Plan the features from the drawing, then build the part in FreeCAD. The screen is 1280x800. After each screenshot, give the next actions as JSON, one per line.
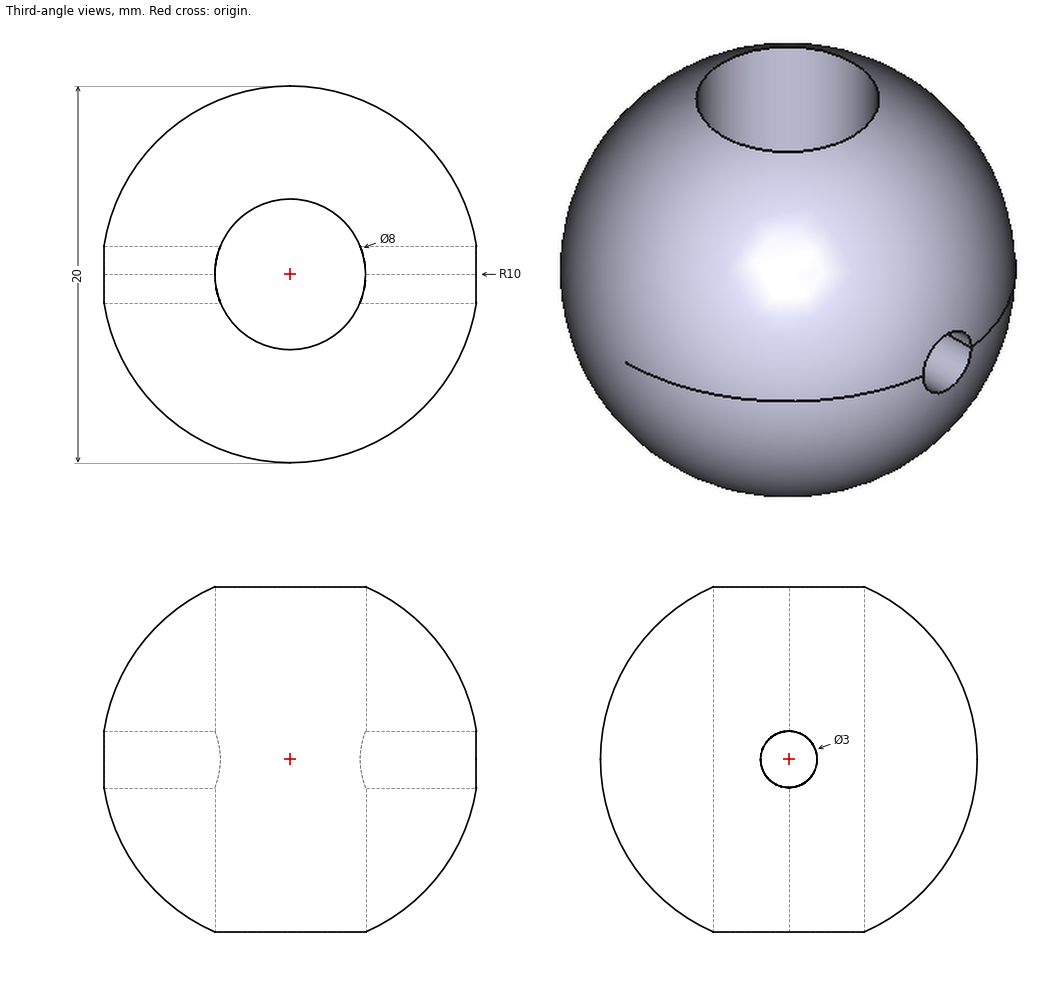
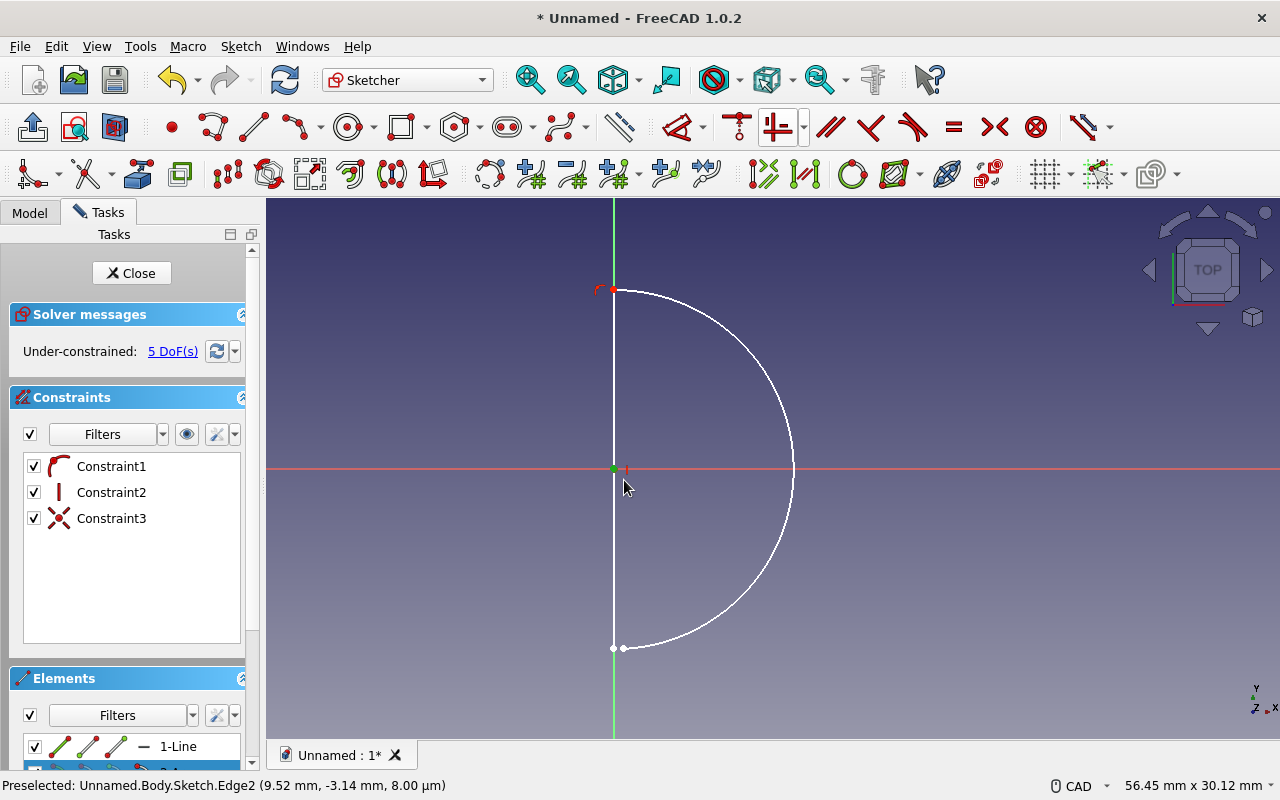
{"action": "left_click", "coordinate": [737, 128]}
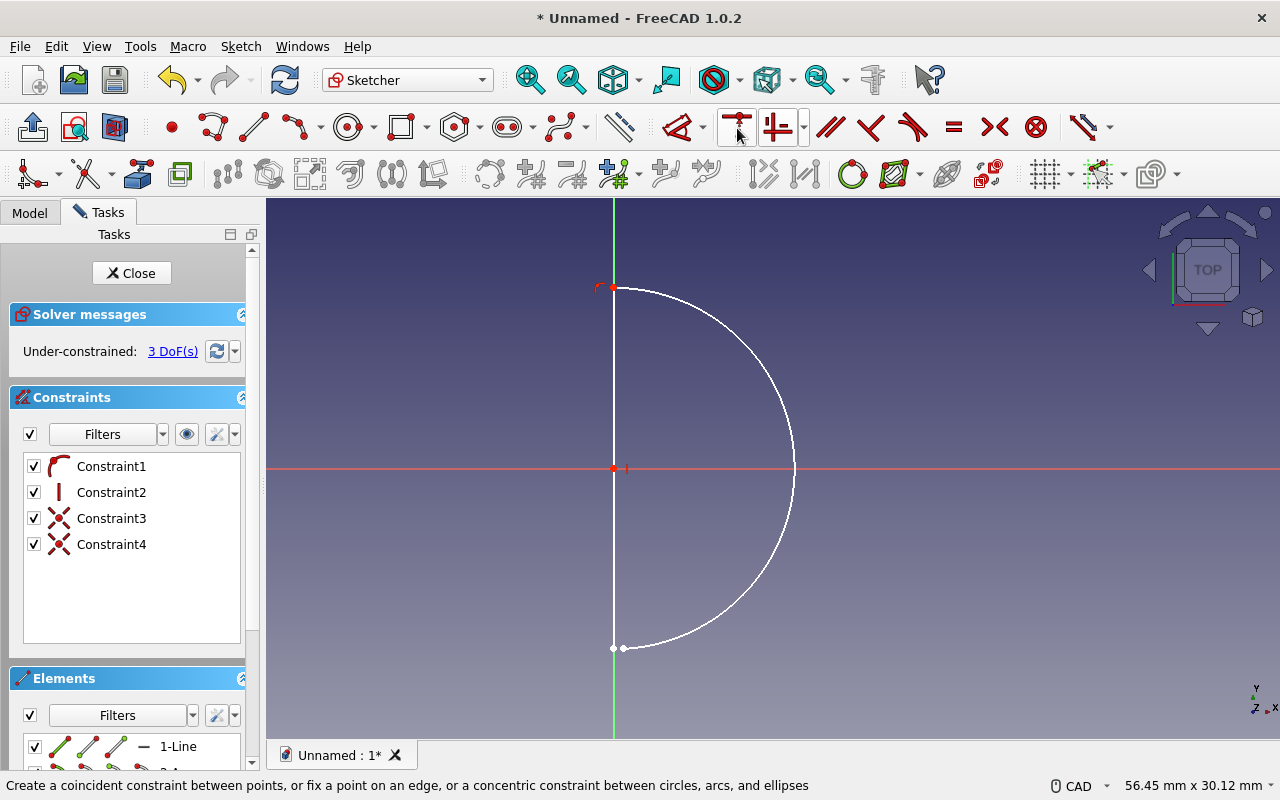
{"action": "left_click", "coordinate": [764, 570]}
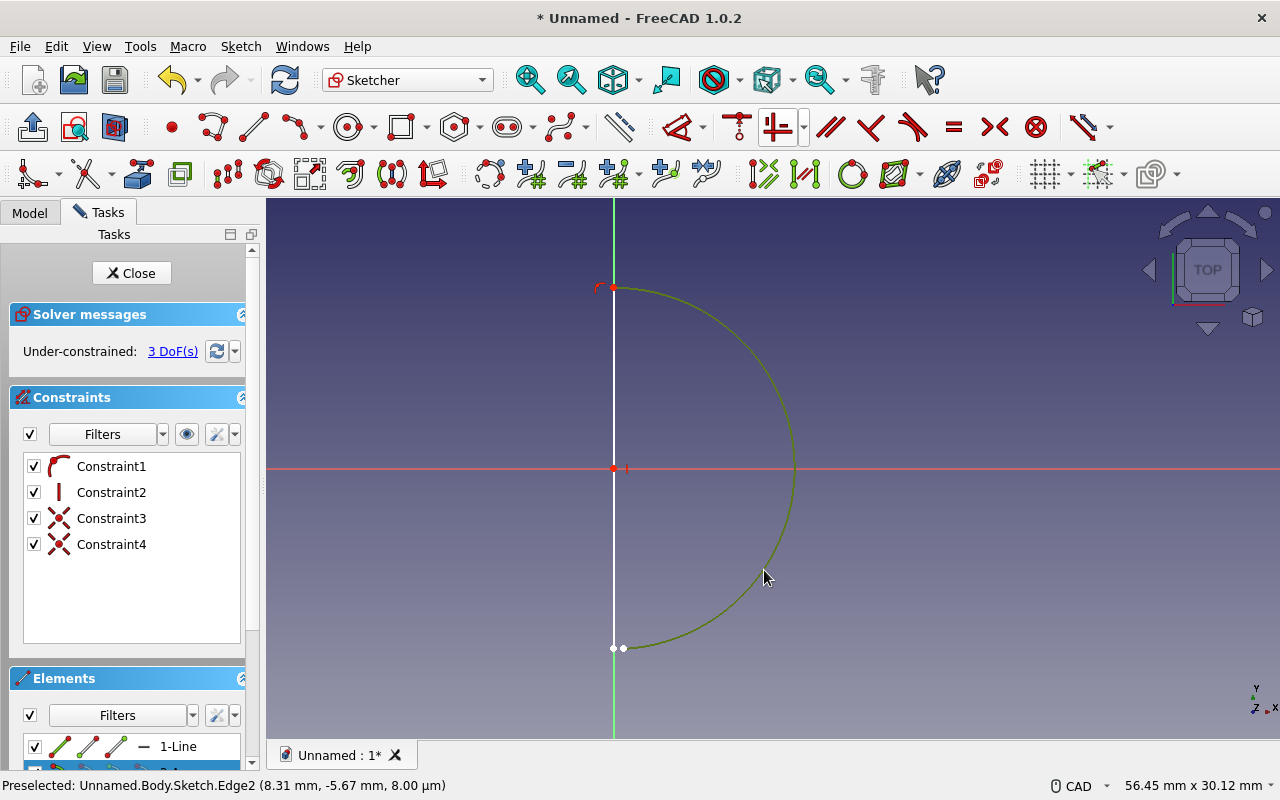
{"action": "left_click", "coordinate": [702, 128]}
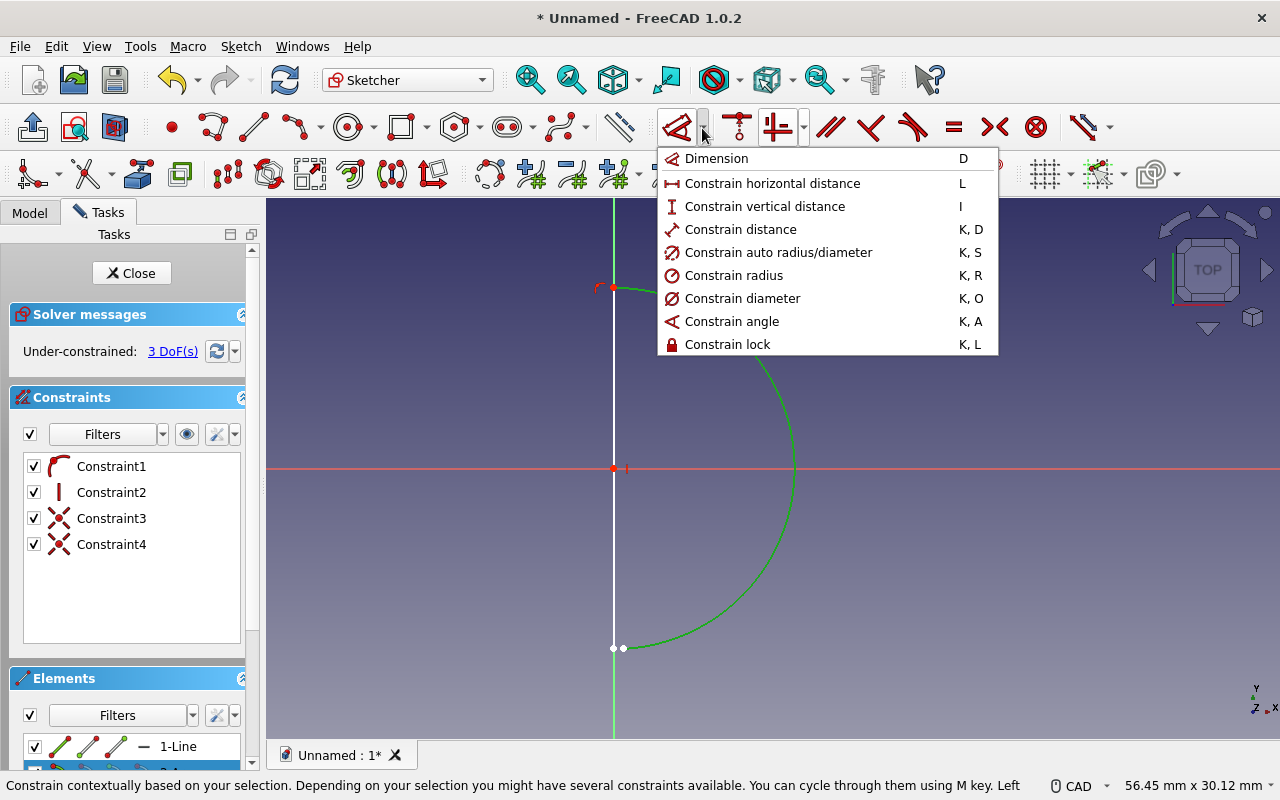
{"action": "left_click", "coordinate": [828, 276]}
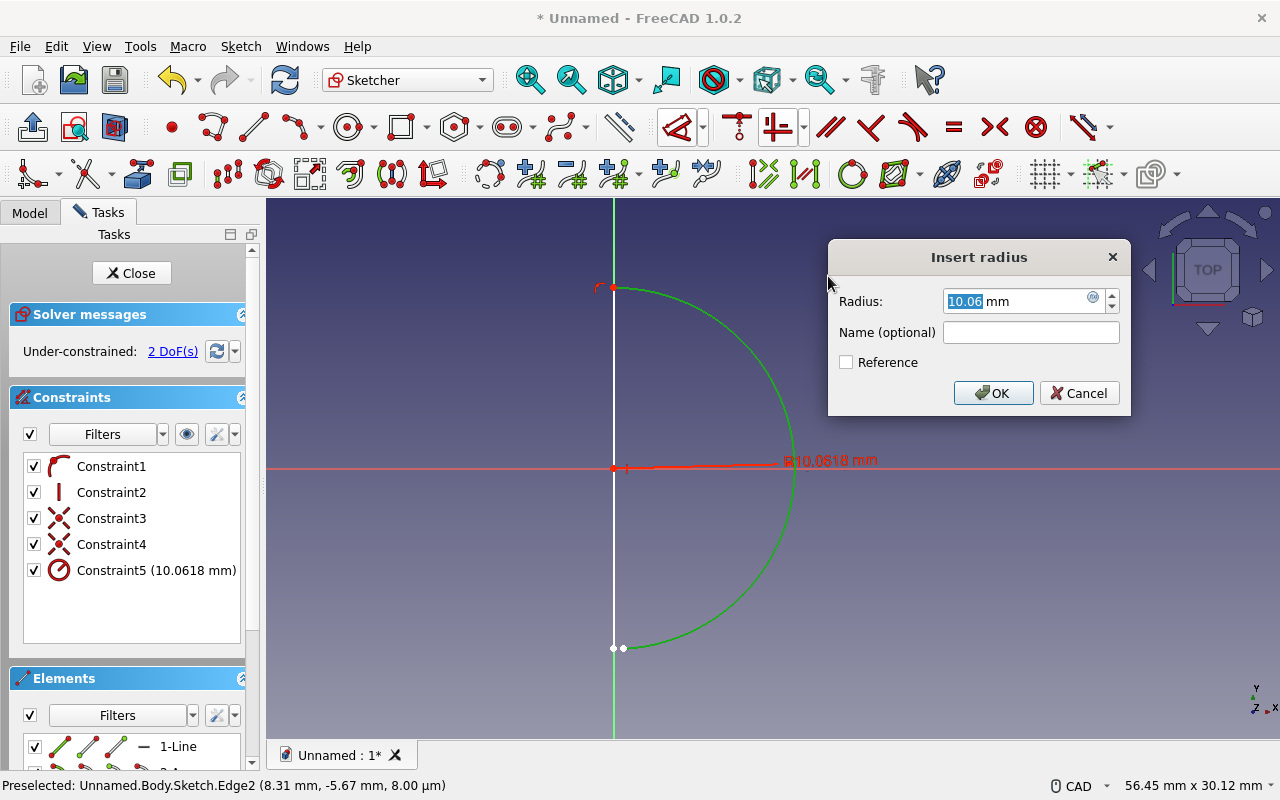
{"action": "type", "text": "10"}
{"action": "key", "text": "Return"}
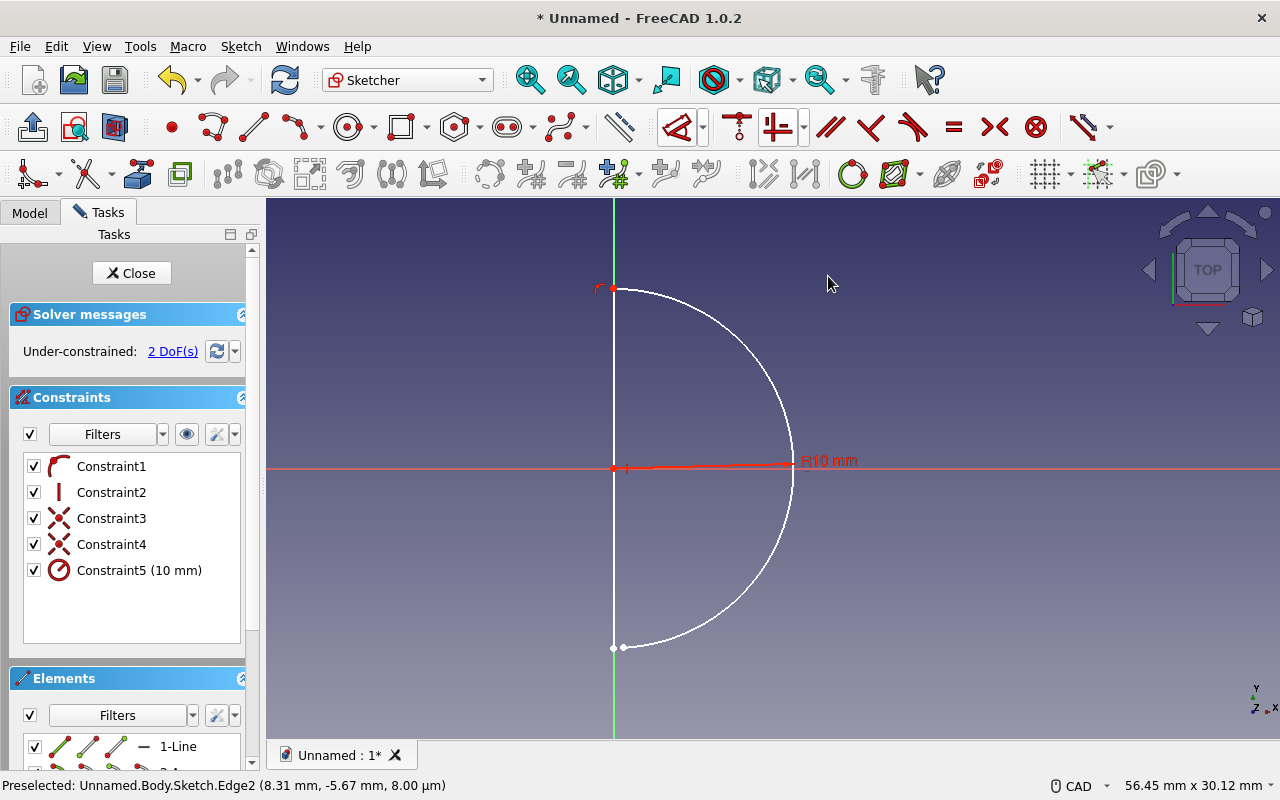
{"action": "left_click", "coordinate": [623, 648]}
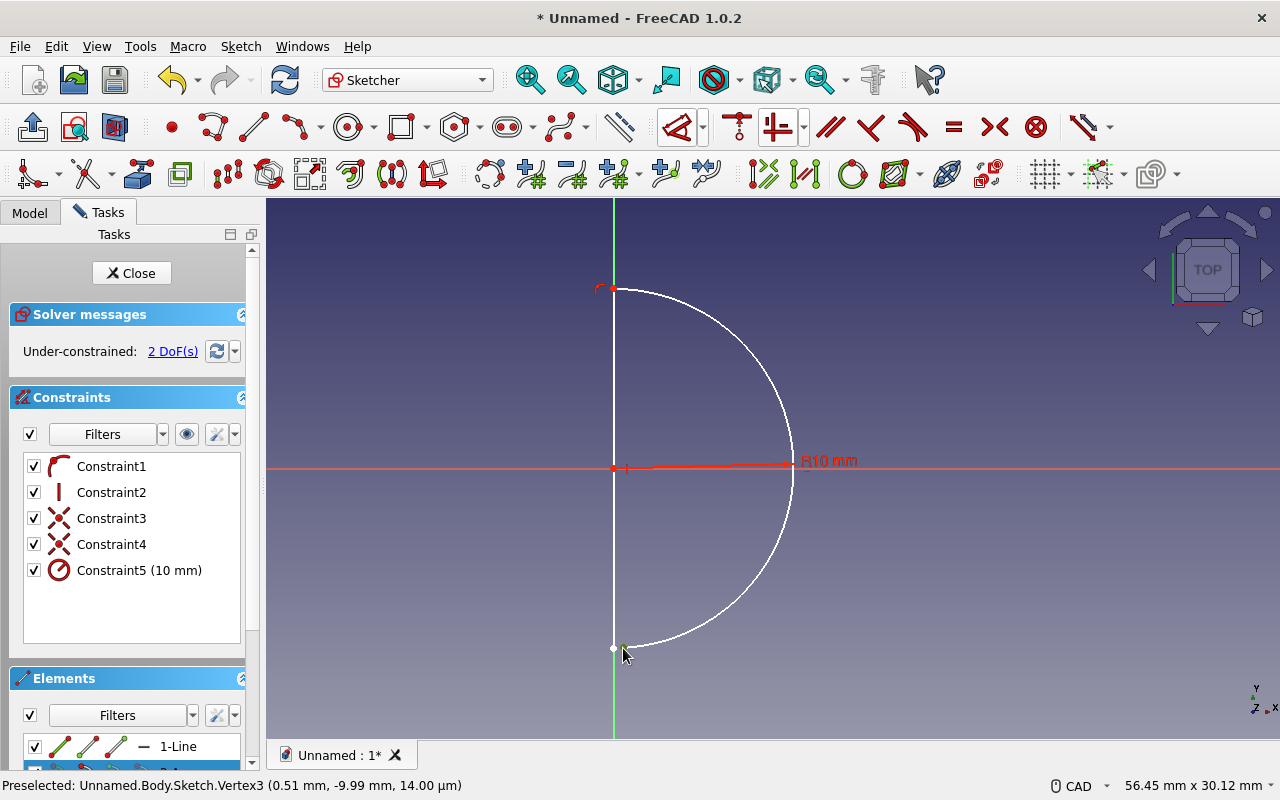
{"action": "left_click", "coordinate": [614, 261]}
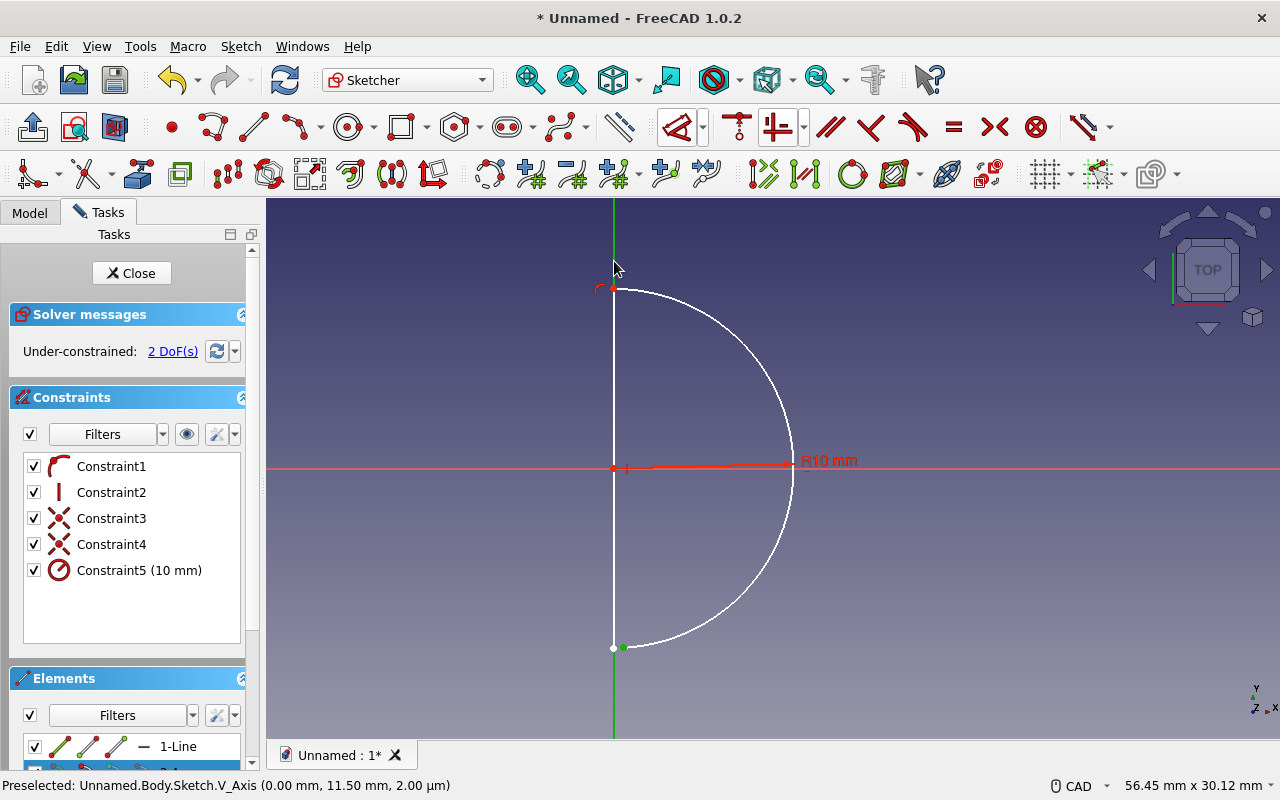
{"action": "left_click", "coordinate": [737, 128]}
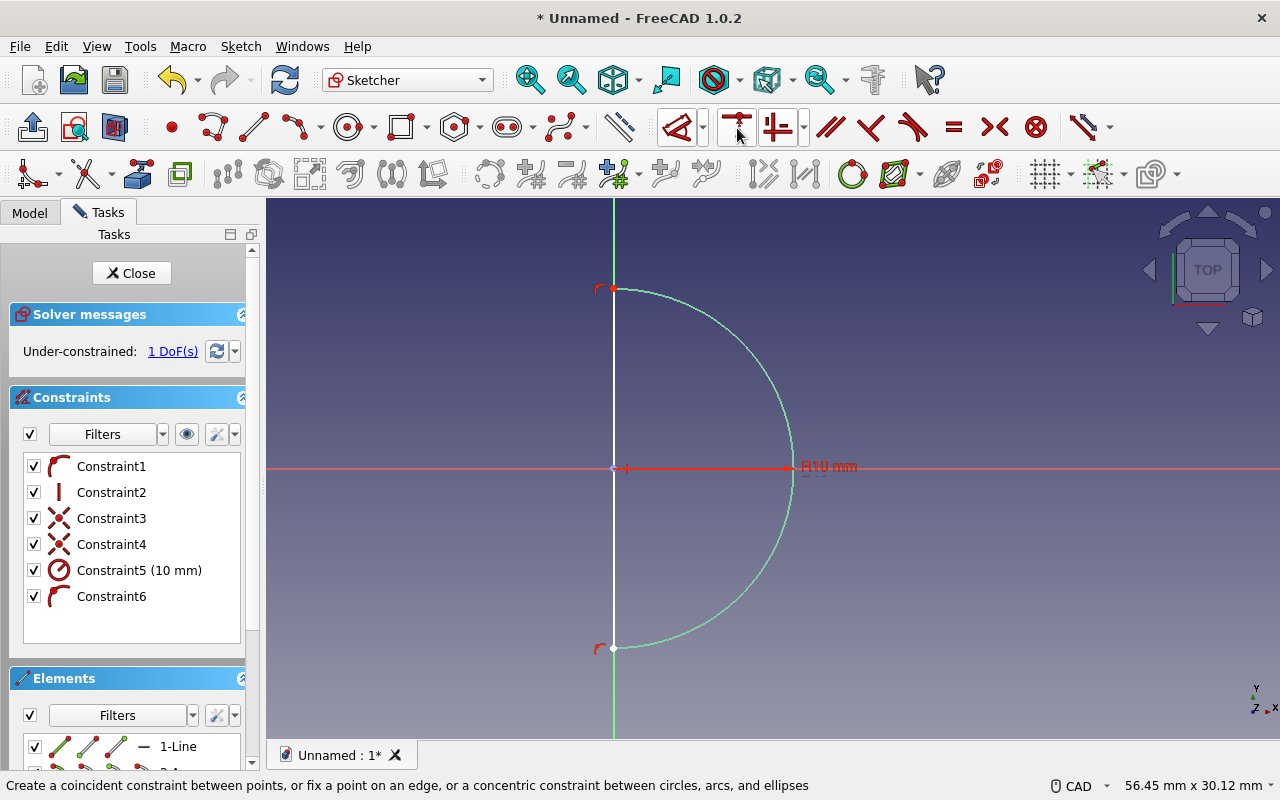
{"action": "left_click", "coordinate": [614, 397]}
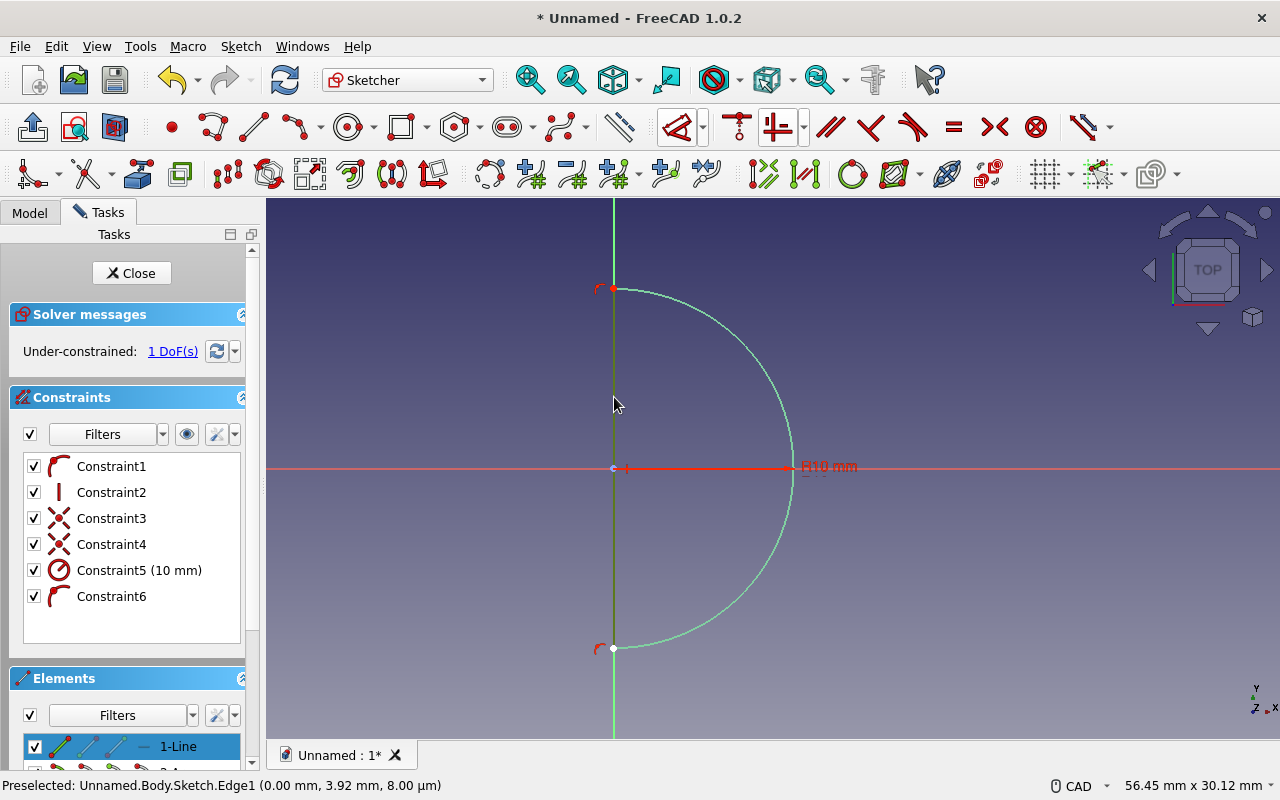
{"action": "key", "text": "i"}